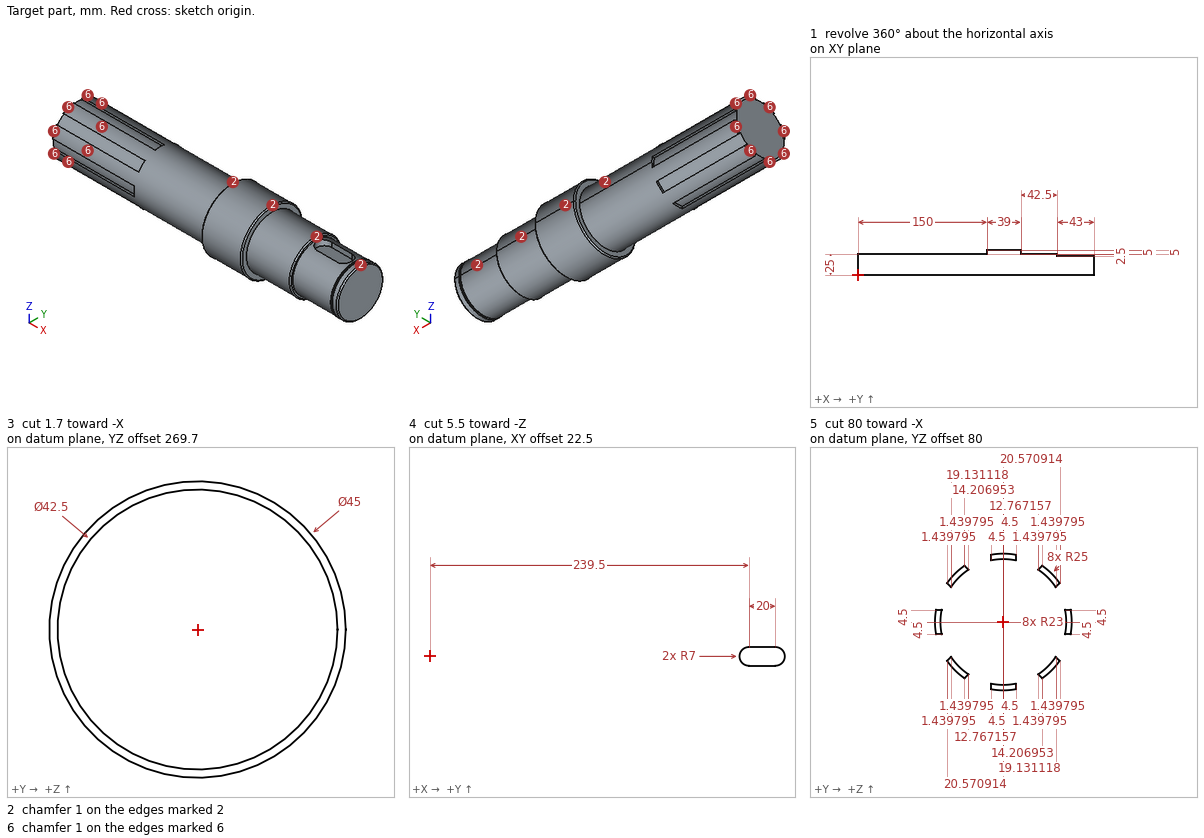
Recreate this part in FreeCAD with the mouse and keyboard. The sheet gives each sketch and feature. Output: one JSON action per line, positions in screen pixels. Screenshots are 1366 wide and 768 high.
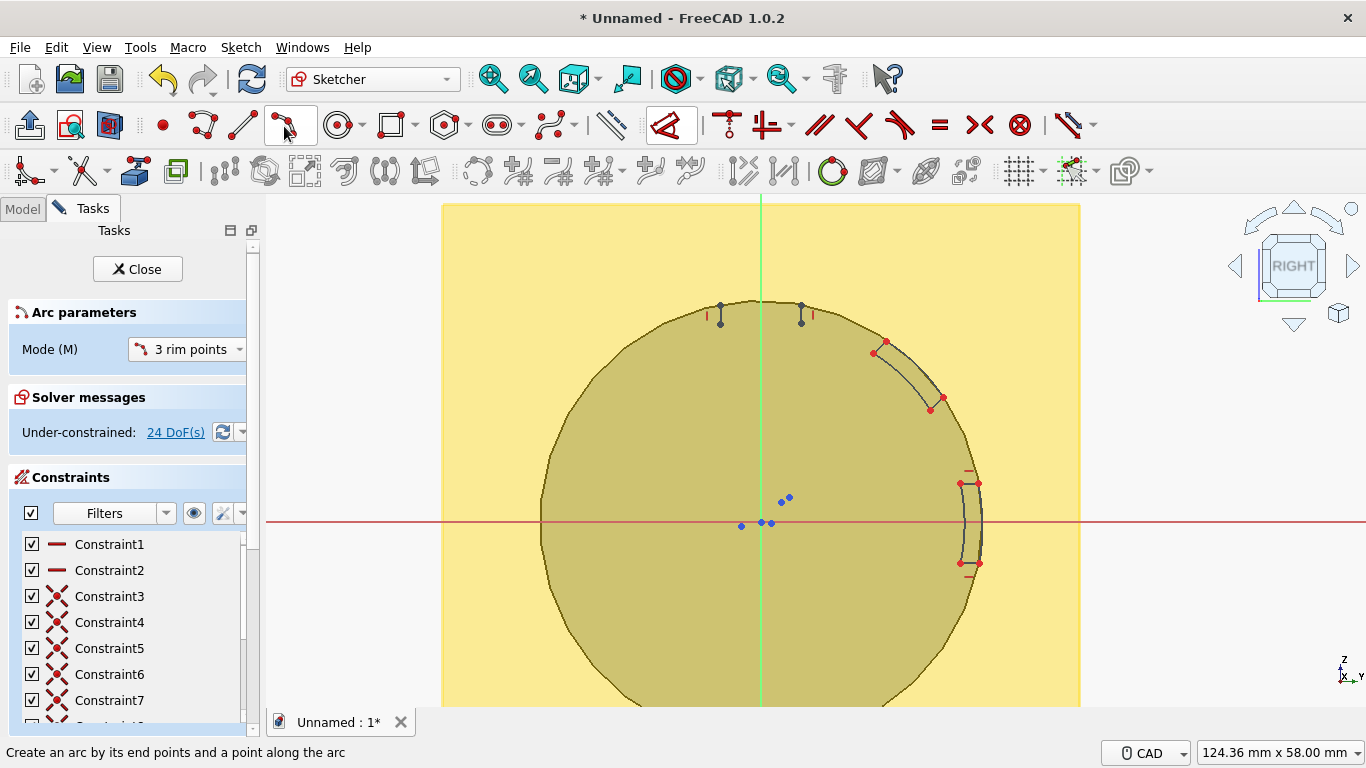
{"action": "scroll", "coordinate": [721, 305], "scroll_direction": "up", "scroll_amount": 3}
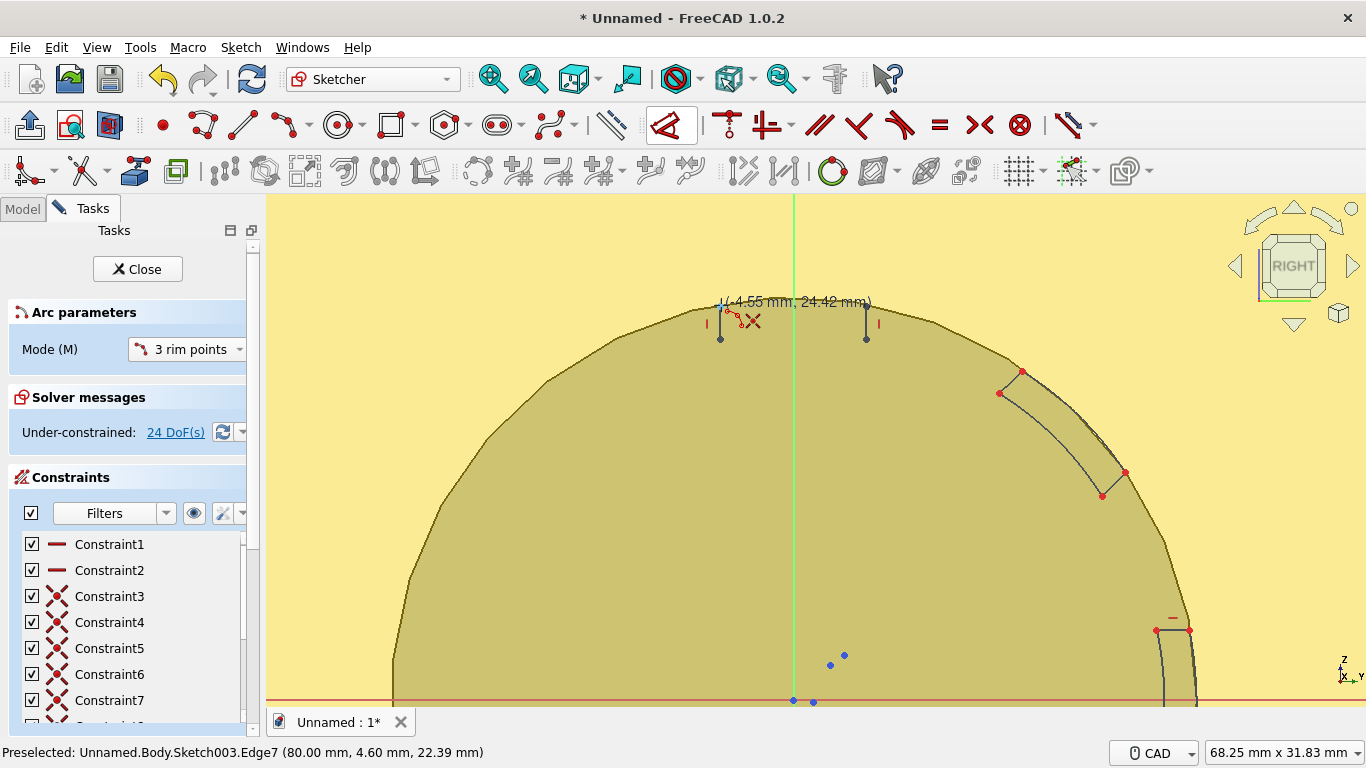
{"action": "left_click", "coordinate": [720, 307]}
{"action": "left_click", "coordinate": [866, 307]}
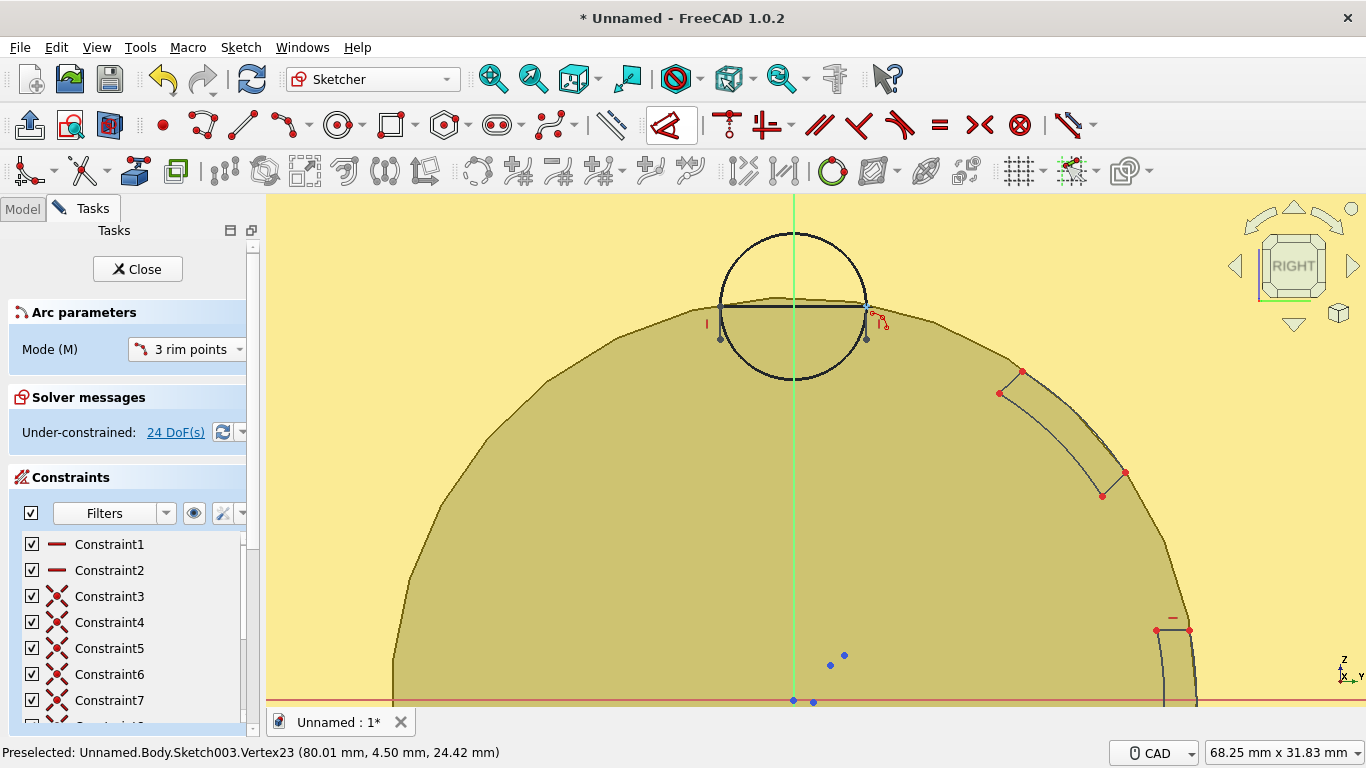
{"action": "scroll", "coordinate": [809, 298], "scroll_direction": "up", "scroll_amount": 5}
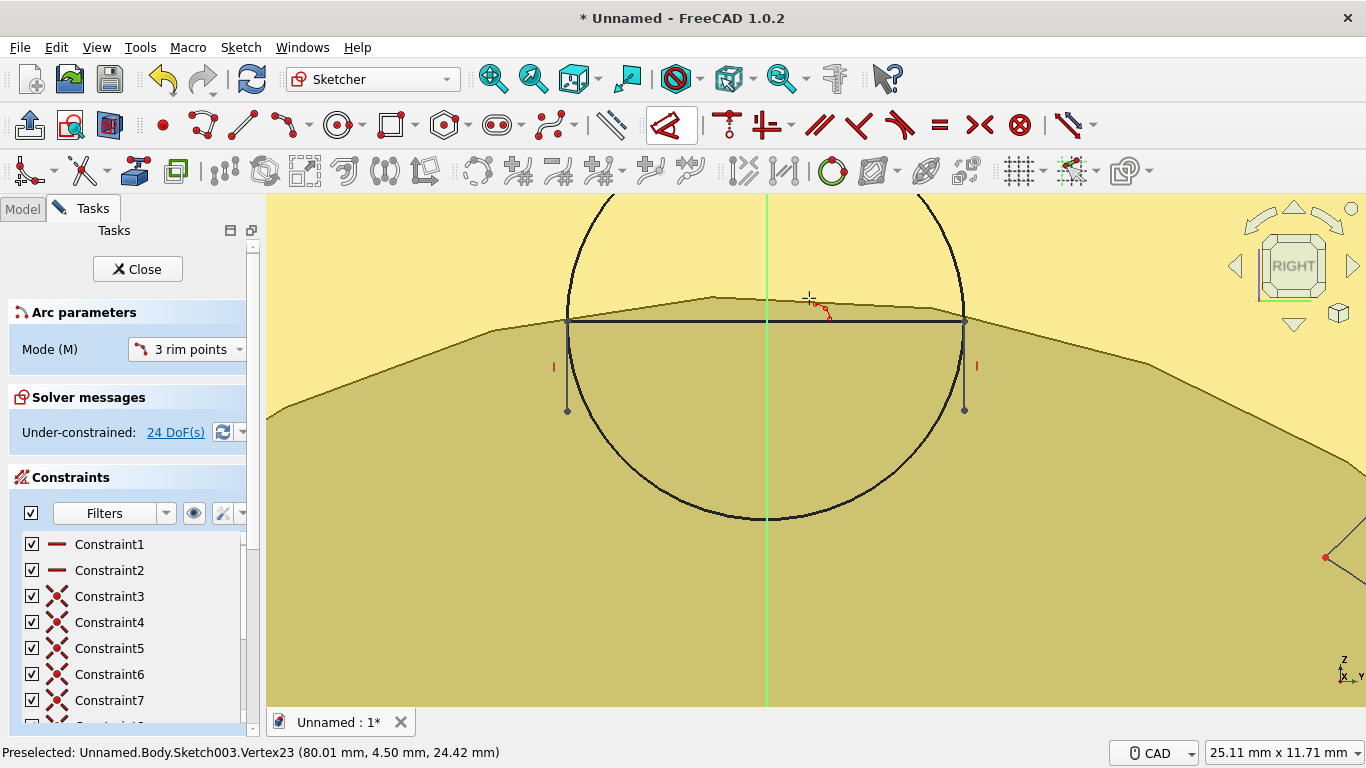
{"action": "left_click", "coordinate": [807, 297]}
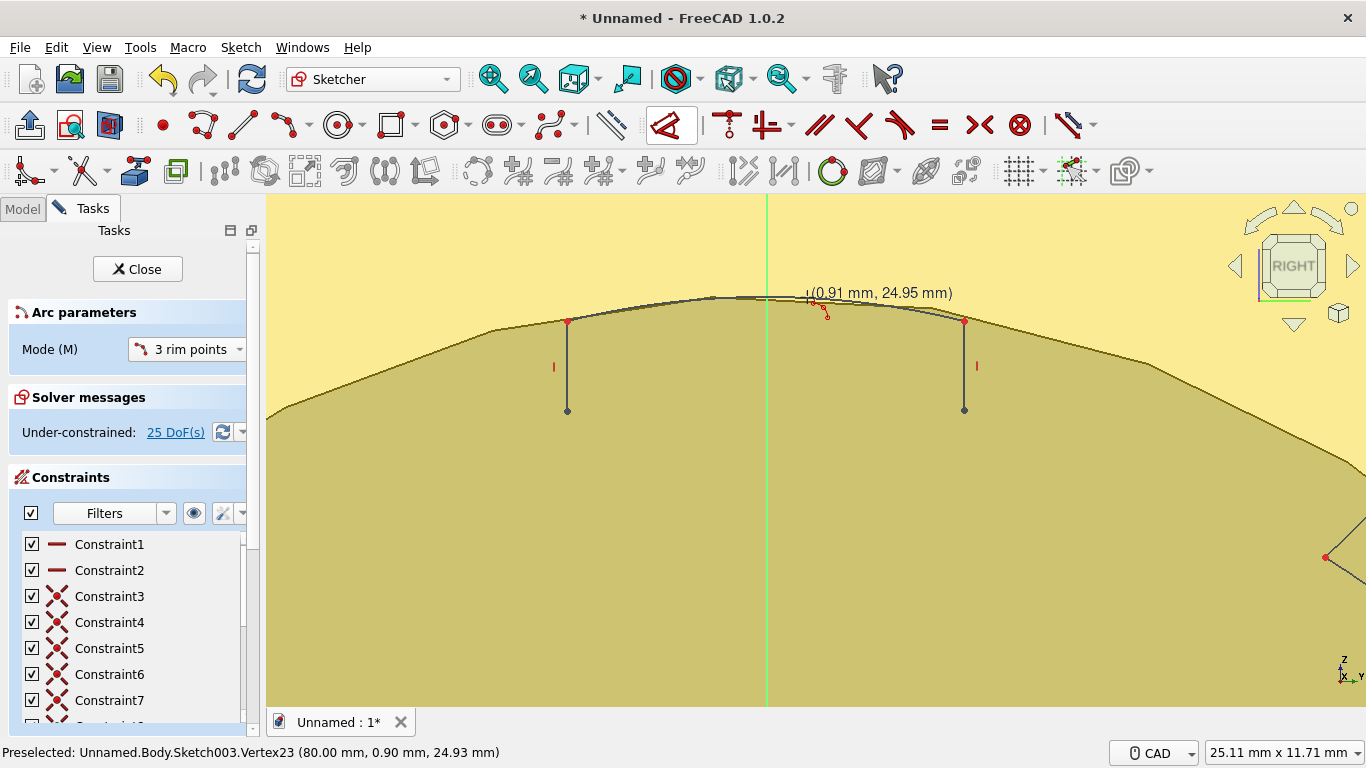
{"action": "left_click", "coordinate": [964, 410]}
{"action": "left_click", "coordinate": [567, 412]}
{"action": "left_click", "coordinate": [807, 384]}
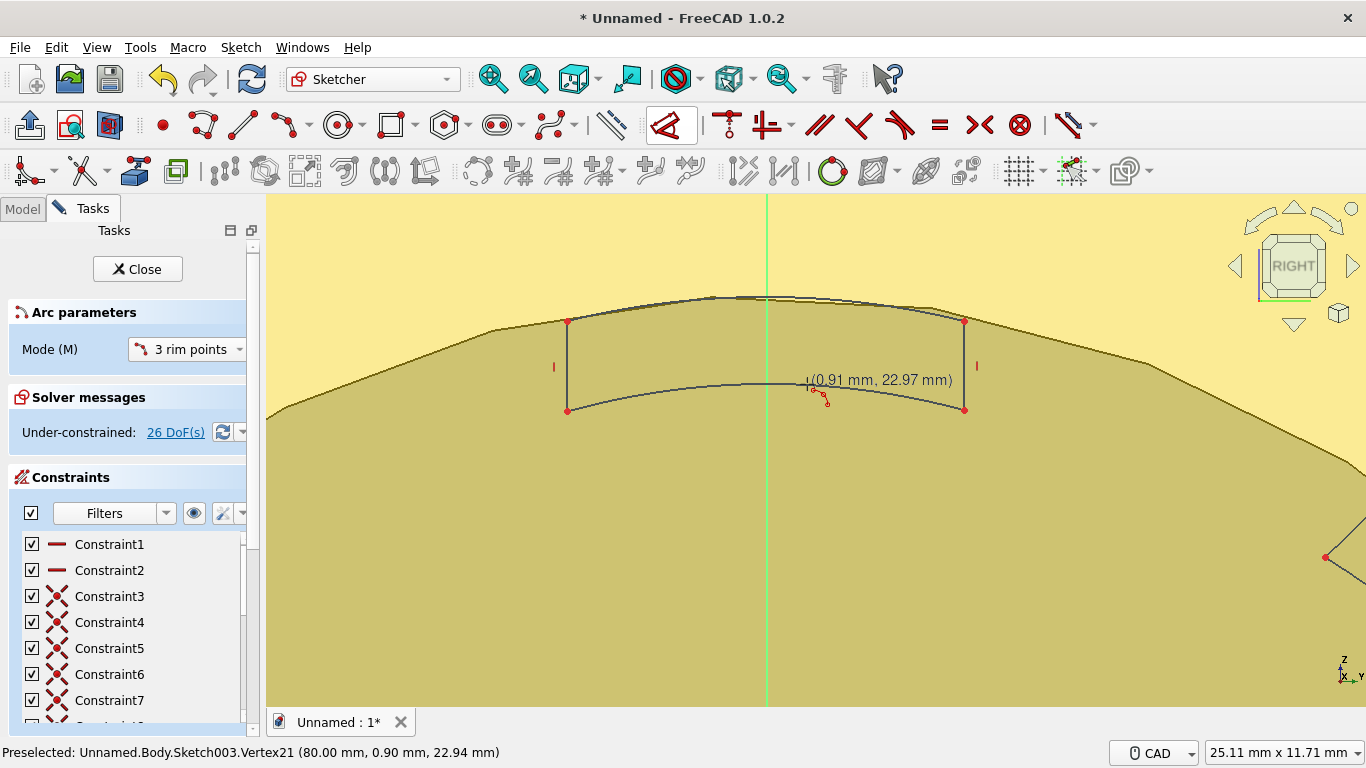
{"action": "left_click", "coordinate": [244, 126]}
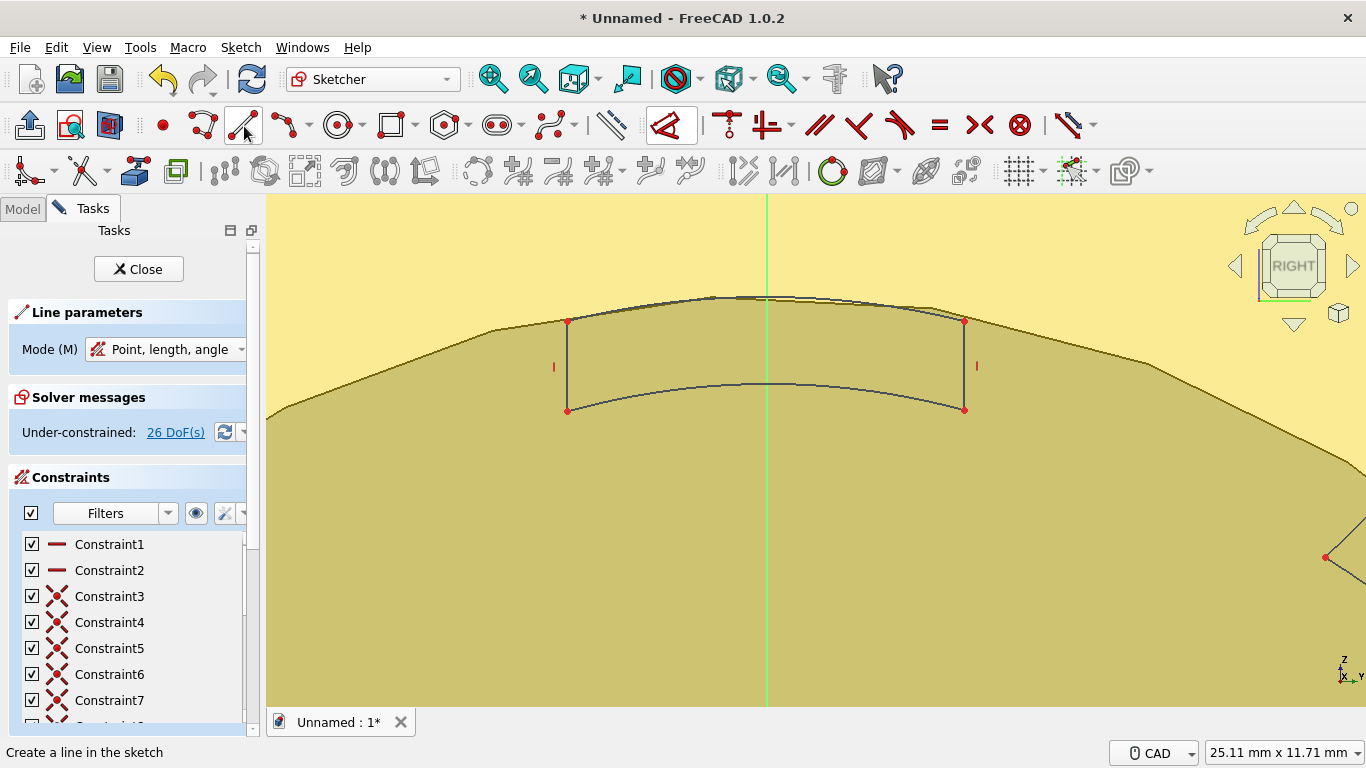
{"action": "scroll", "coordinate": [744, 303], "scroll_direction": "down", "scroll_amount": 10}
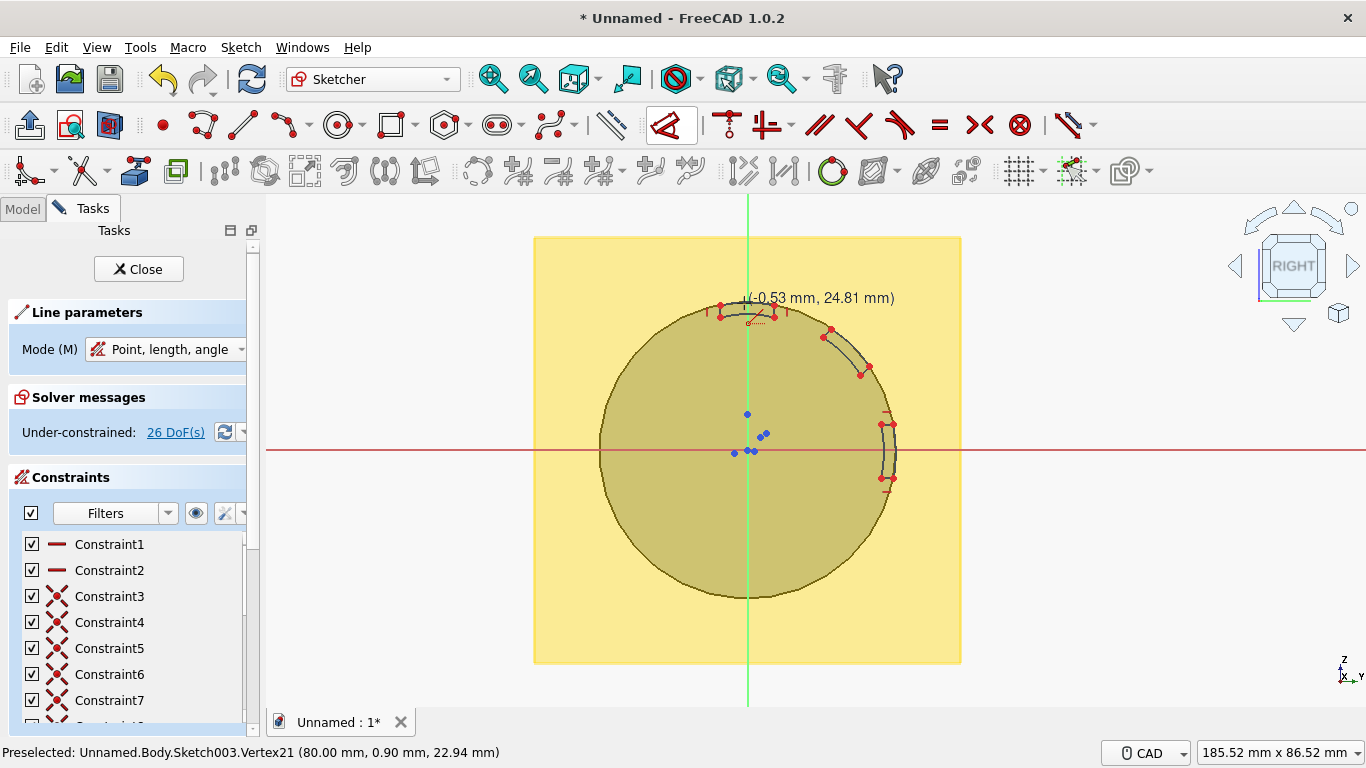
{"action": "left_click", "coordinate": [634, 375]}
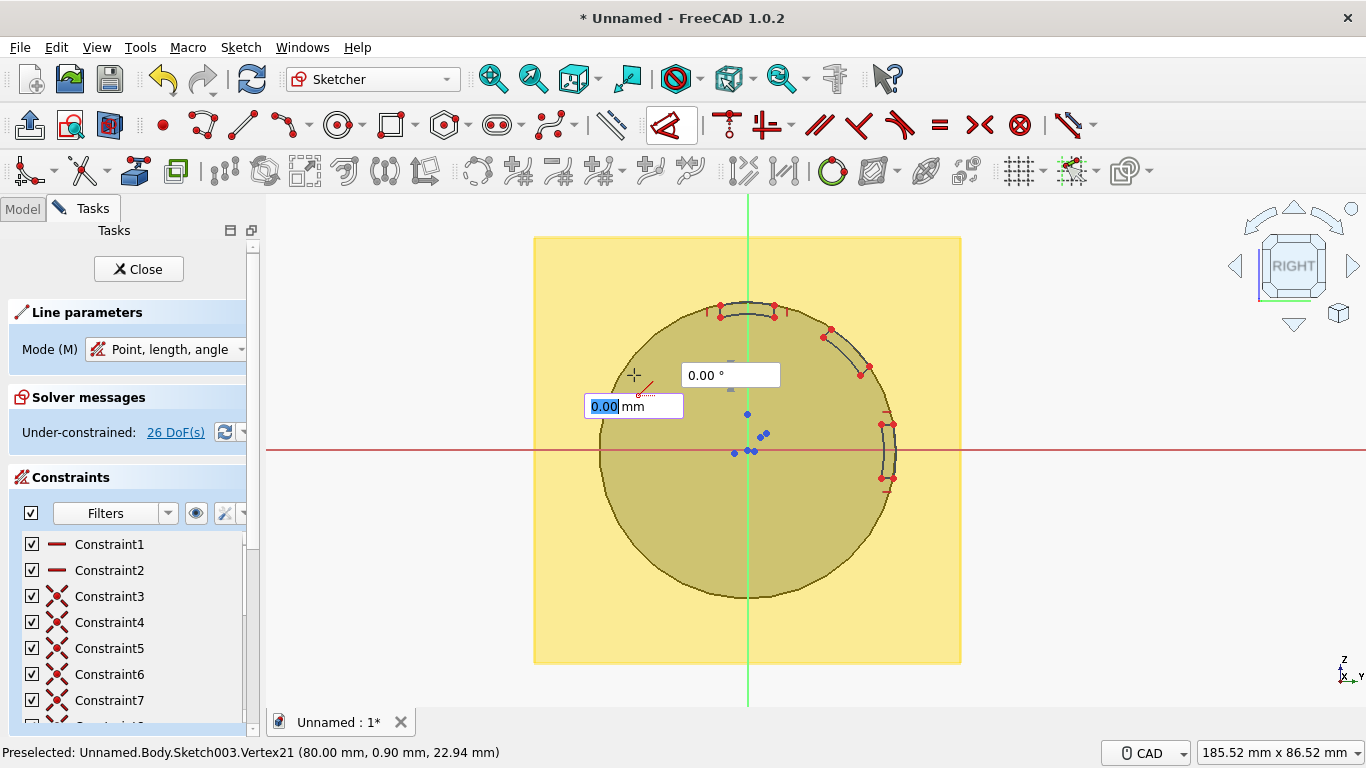
{"action": "scroll", "coordinate": [626, 366], "scroll_direction": "up", "scroll_amount": 2}